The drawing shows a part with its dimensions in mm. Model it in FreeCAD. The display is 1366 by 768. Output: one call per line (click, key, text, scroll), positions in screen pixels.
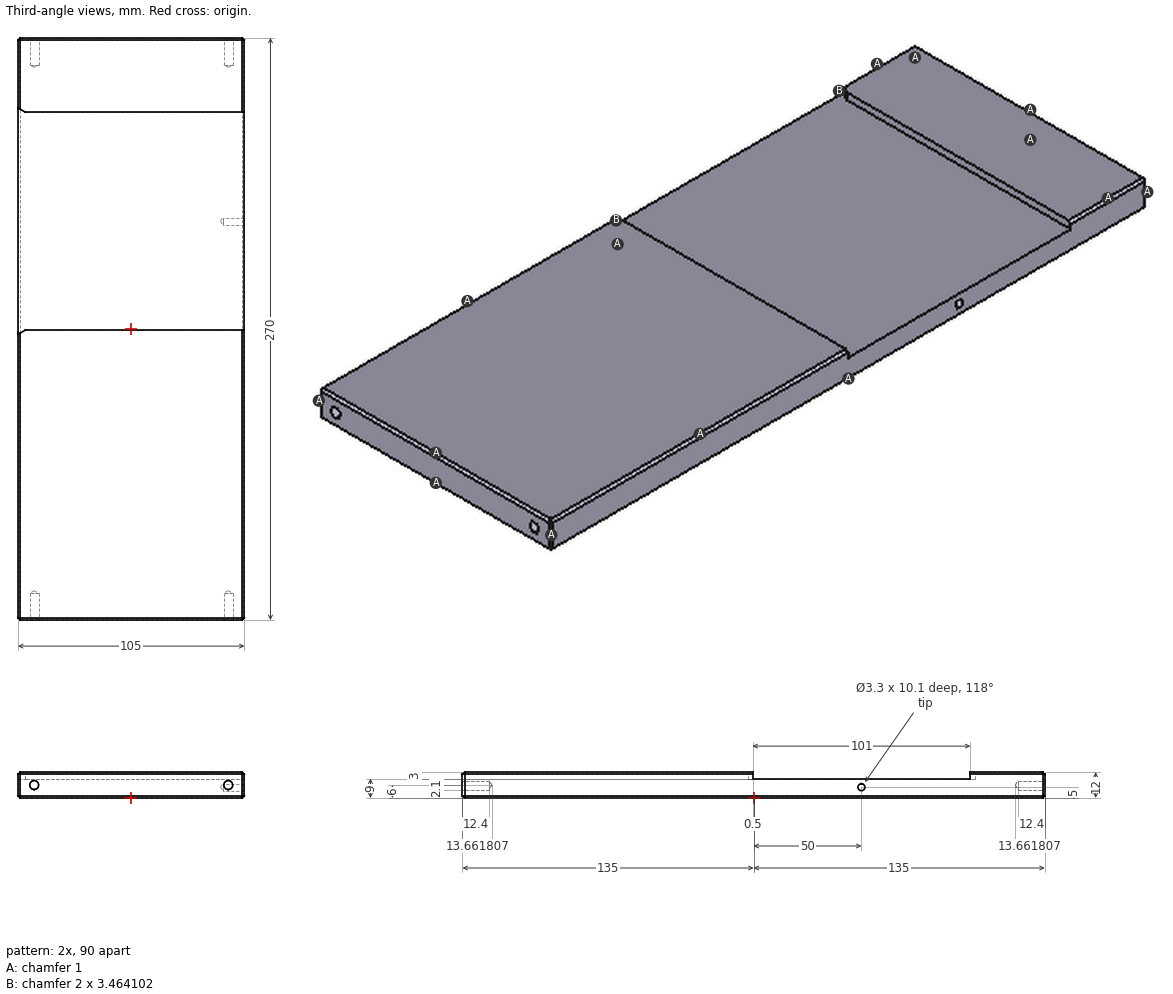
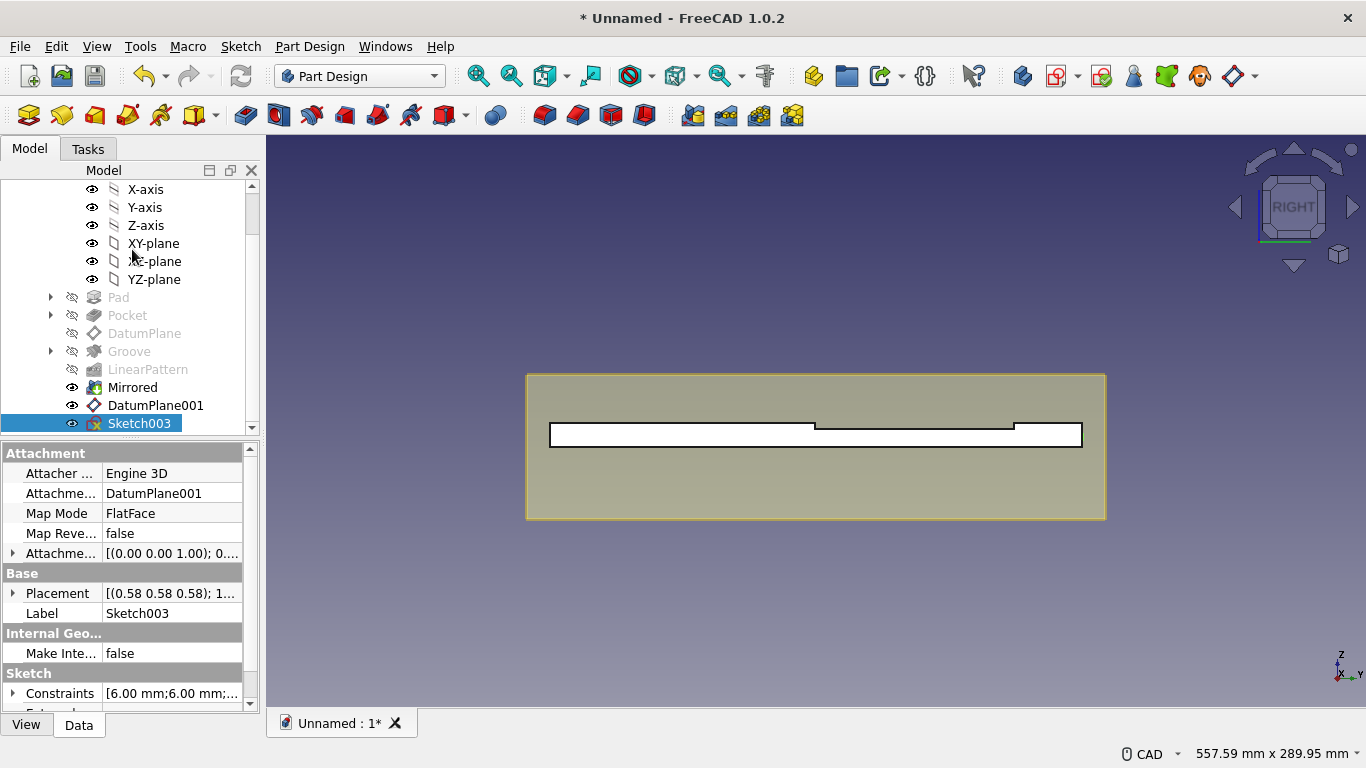
click(312, 116)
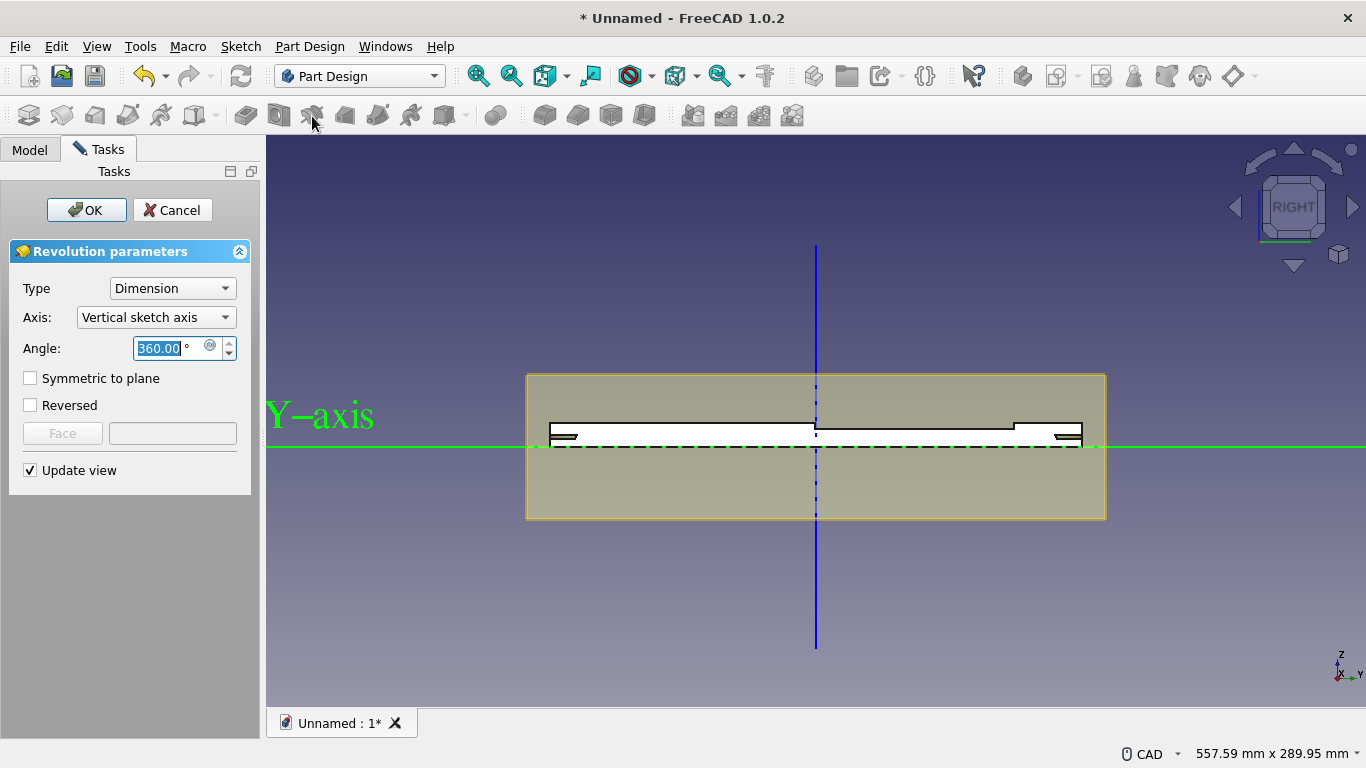
click(157, 318)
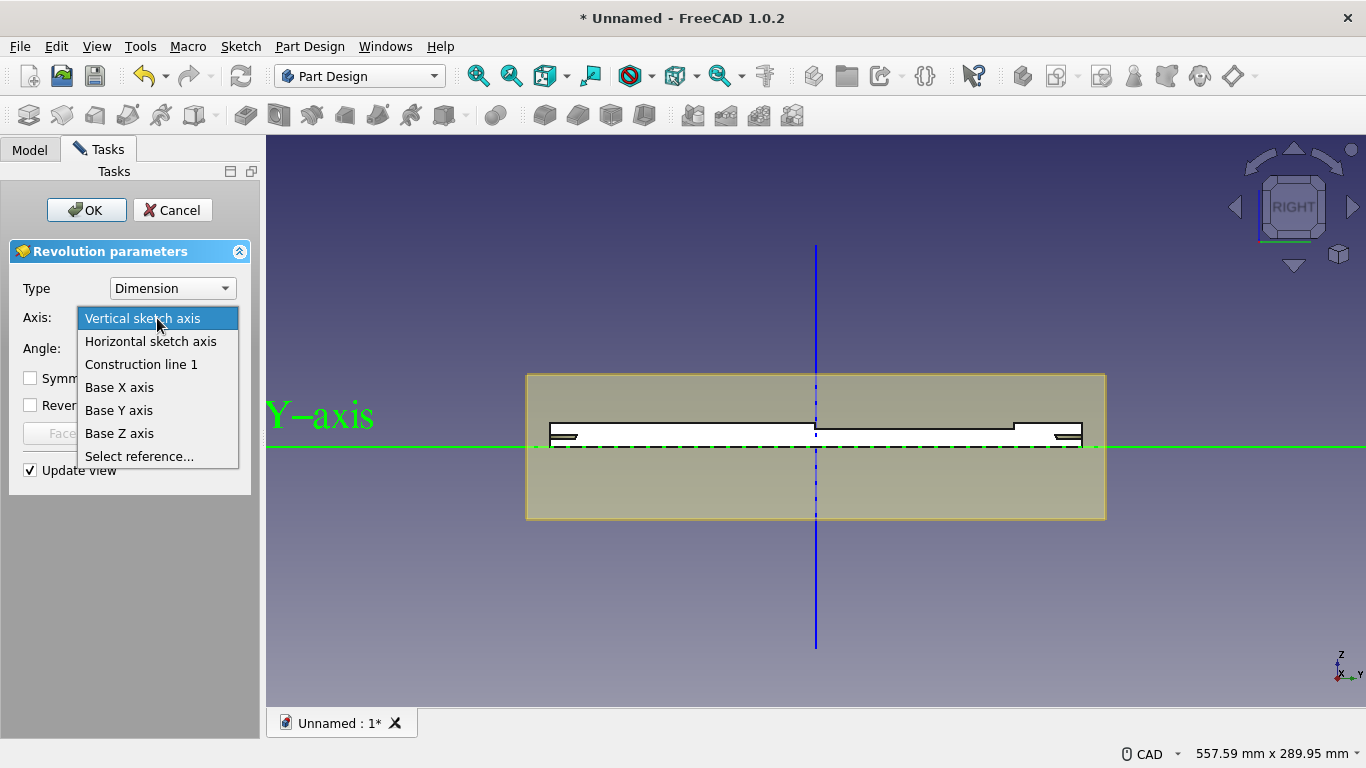
click(156, 364)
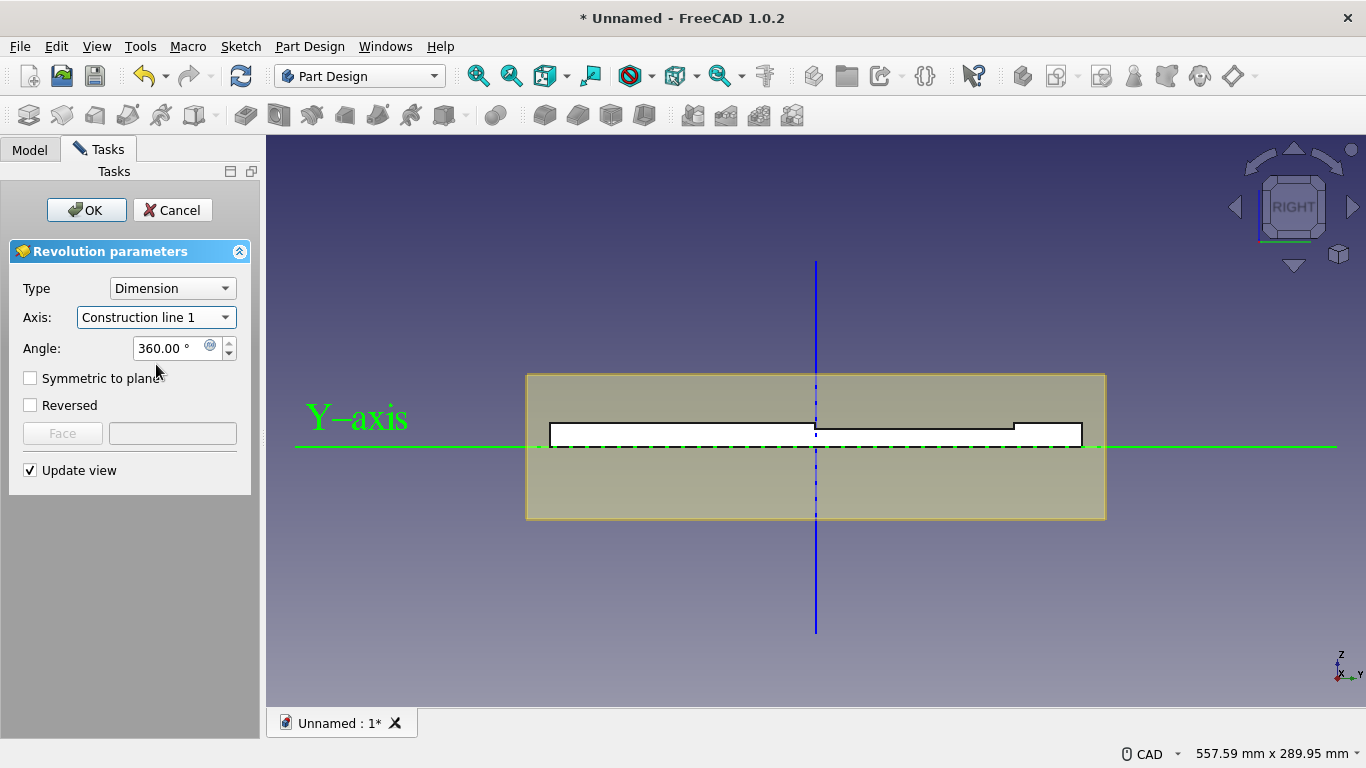
click(87, 210)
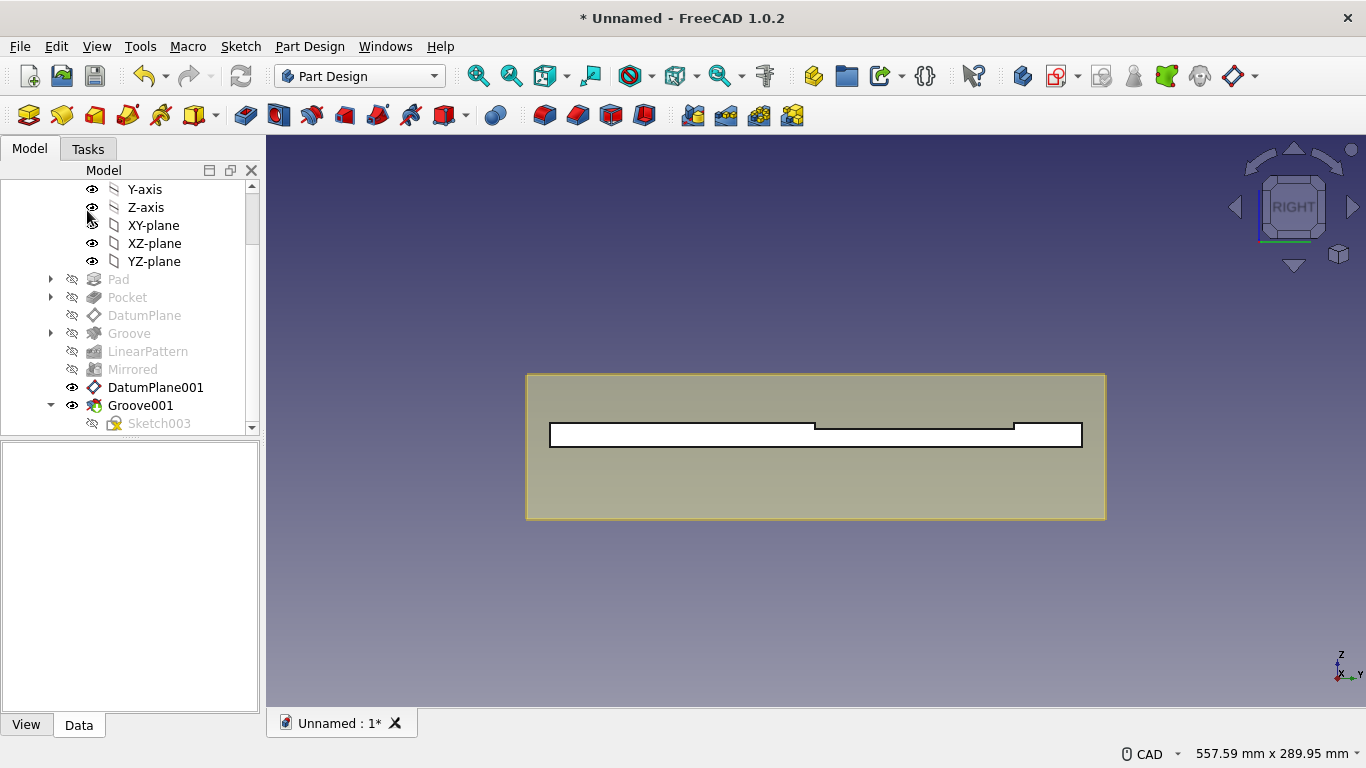
click(117, 387)
key(space)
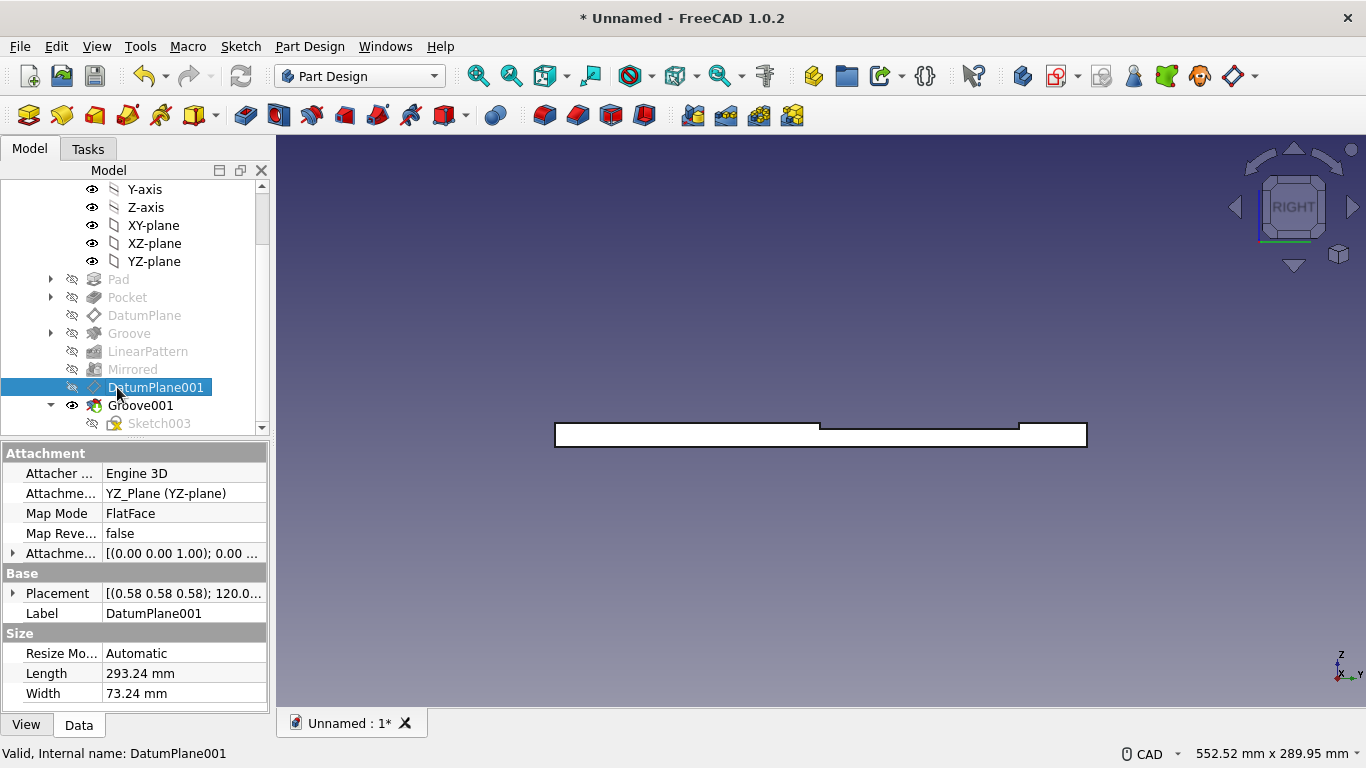
click(1087, 434)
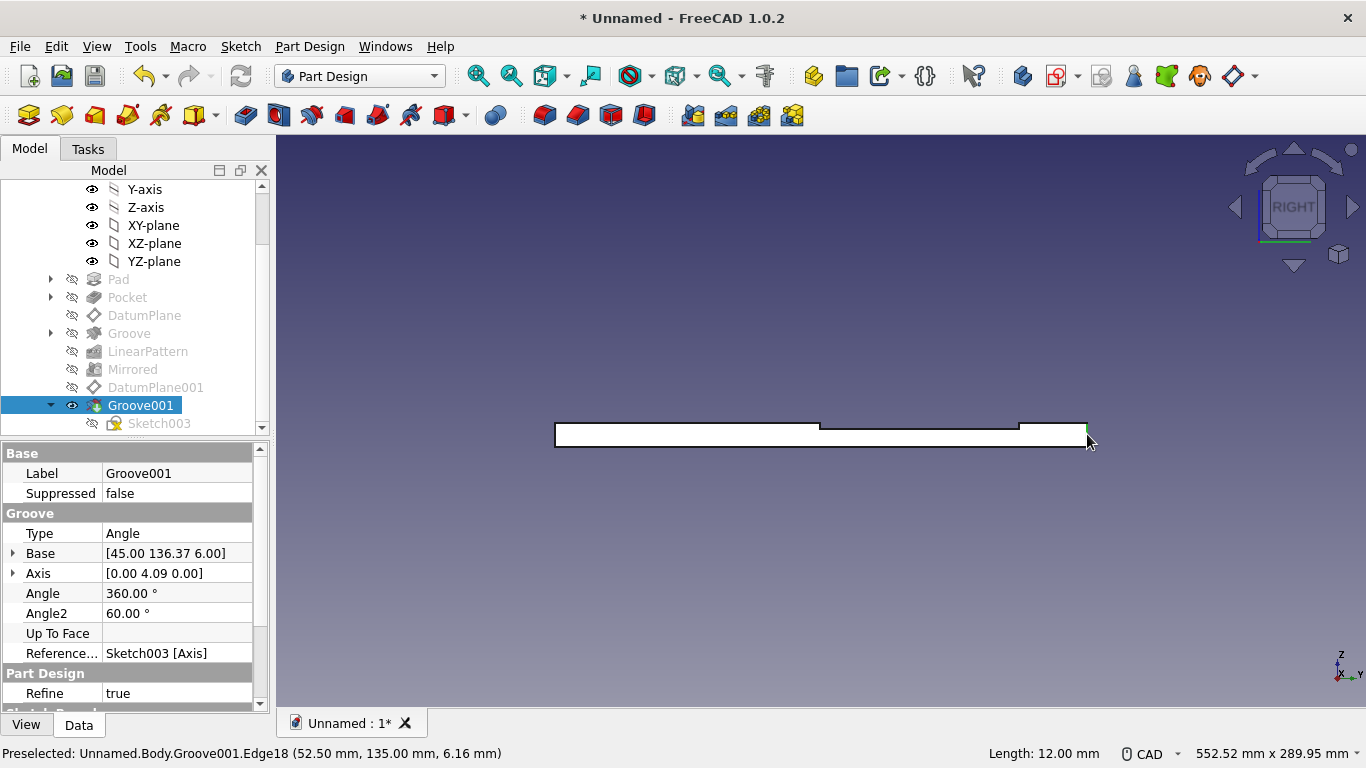
key(0)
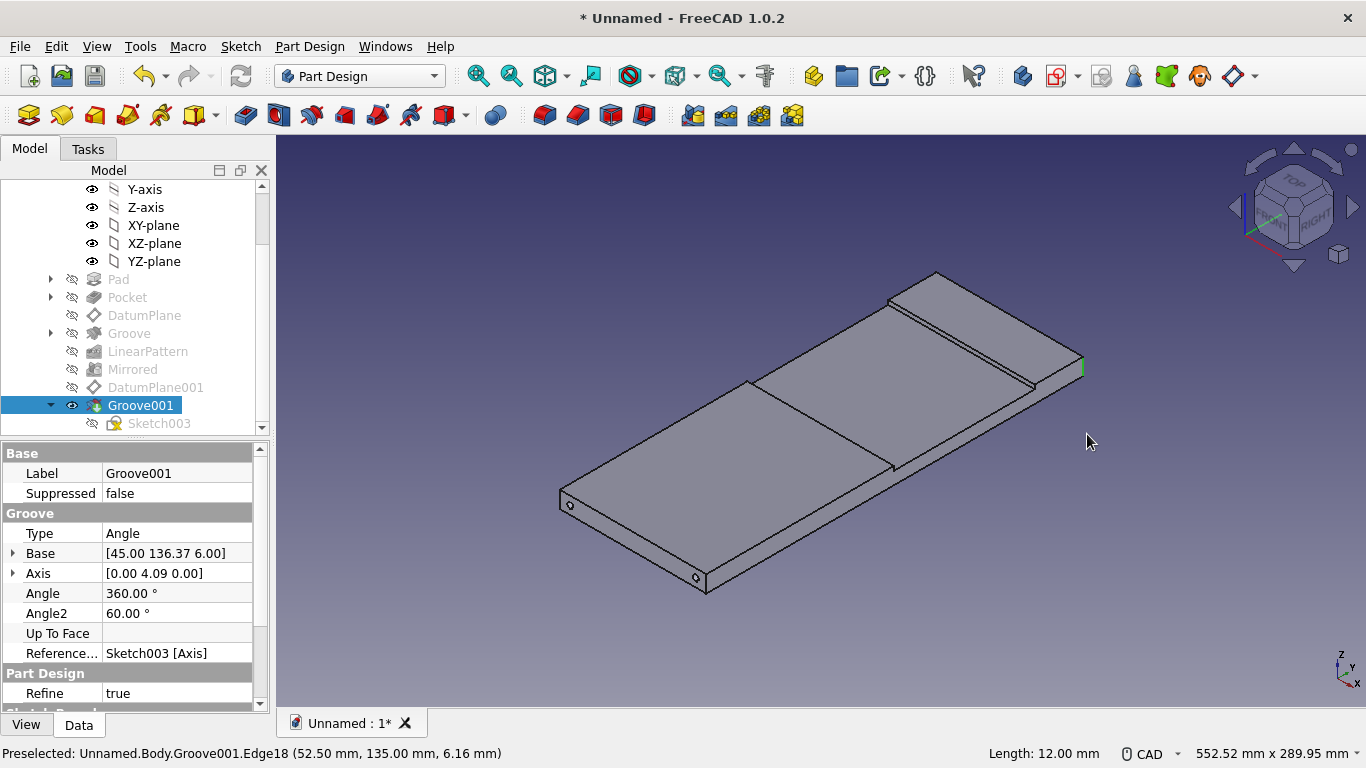
click(633, 531, ctrl)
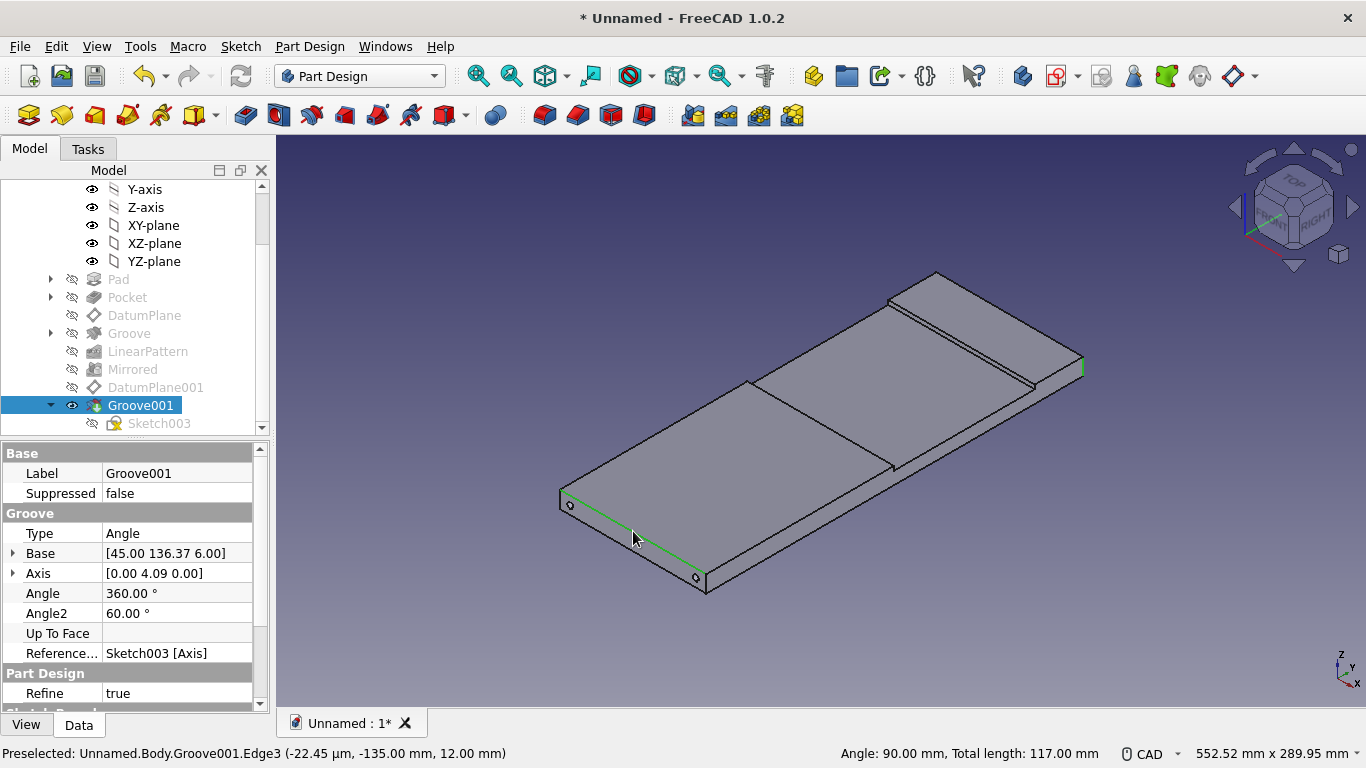
click(1059, 370, ctrl)